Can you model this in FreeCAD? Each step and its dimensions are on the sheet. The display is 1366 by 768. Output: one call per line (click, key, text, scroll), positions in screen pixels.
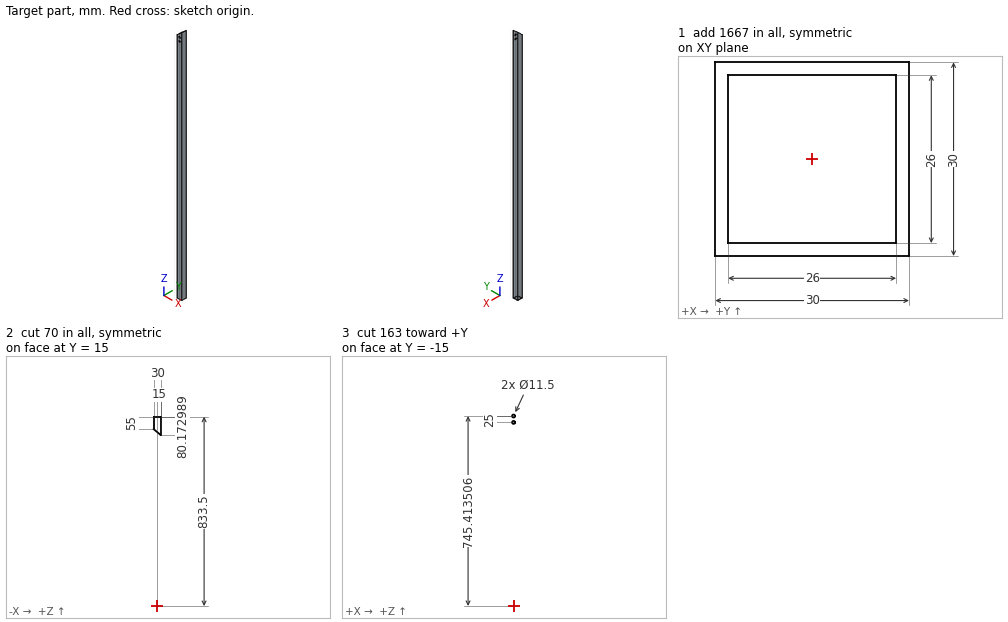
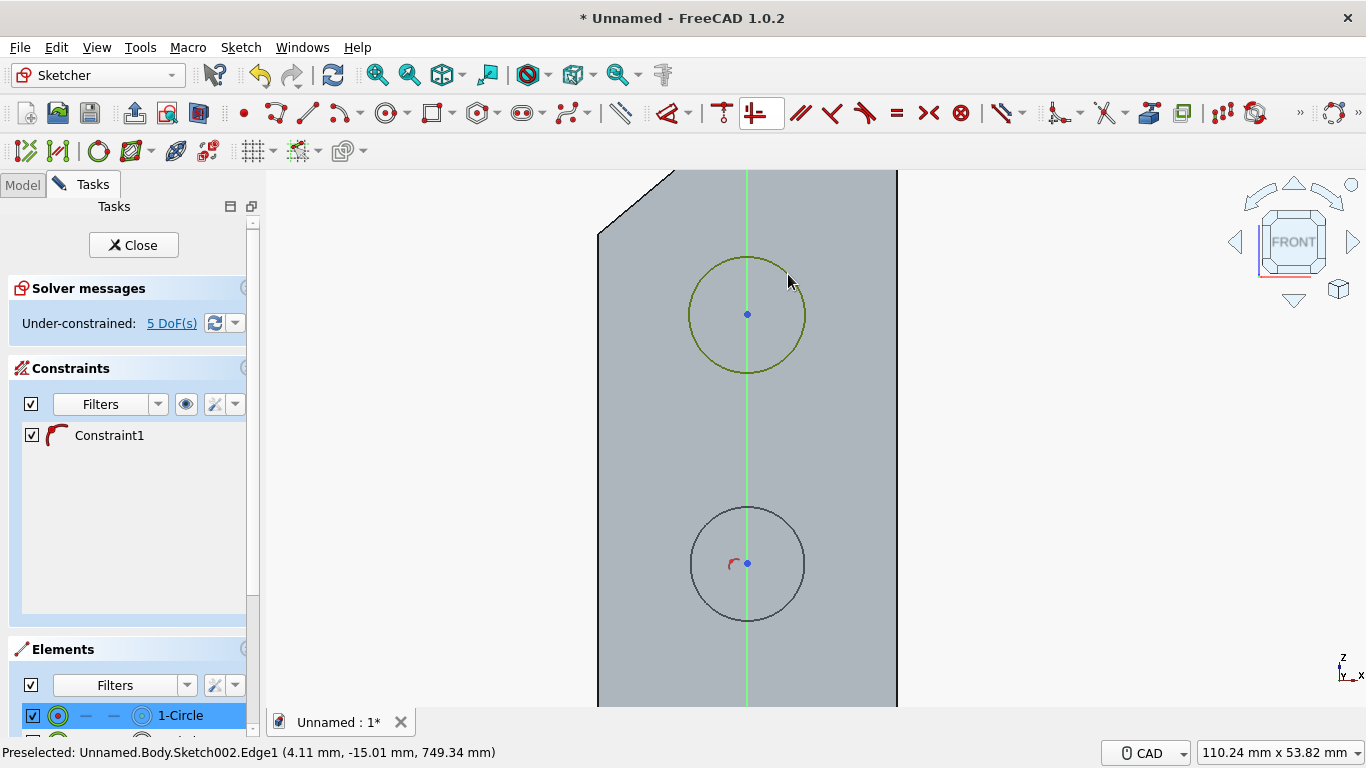
click(788, 524)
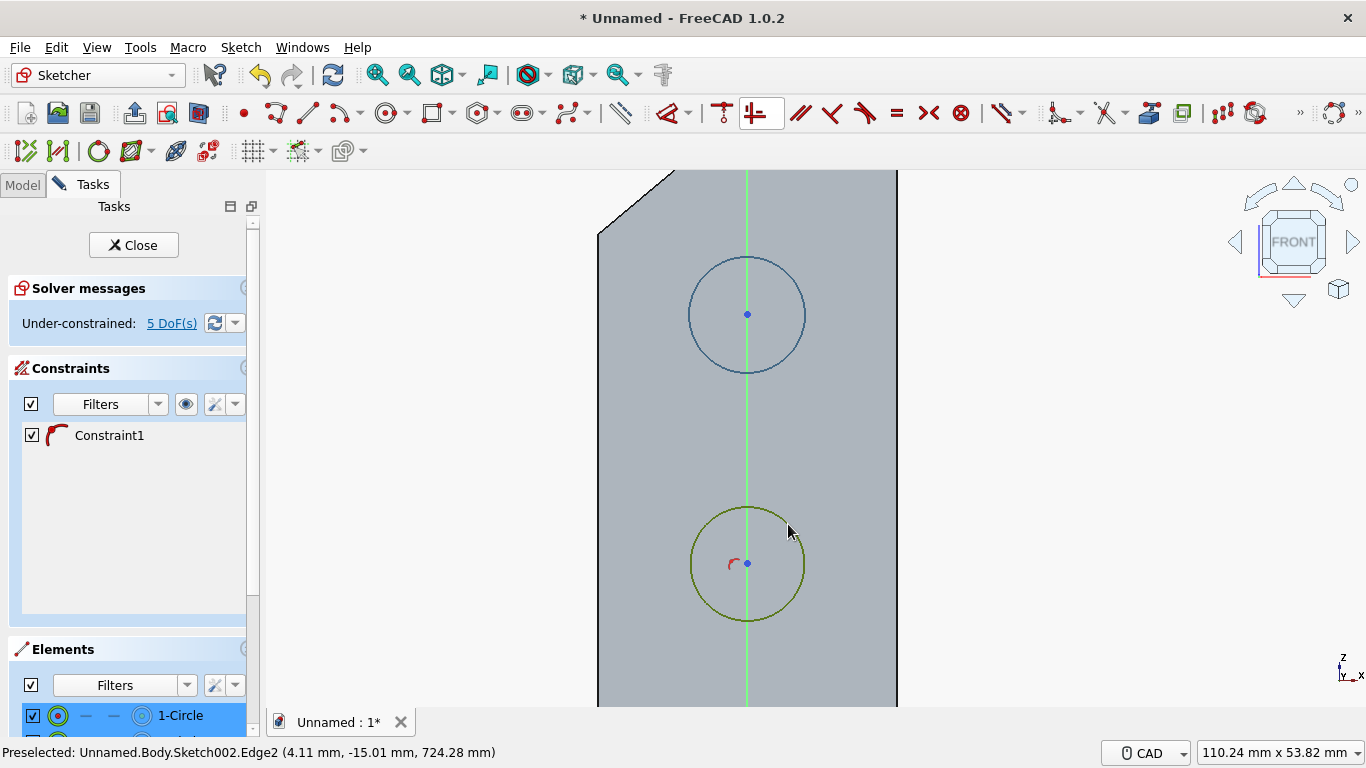
click(898, 114)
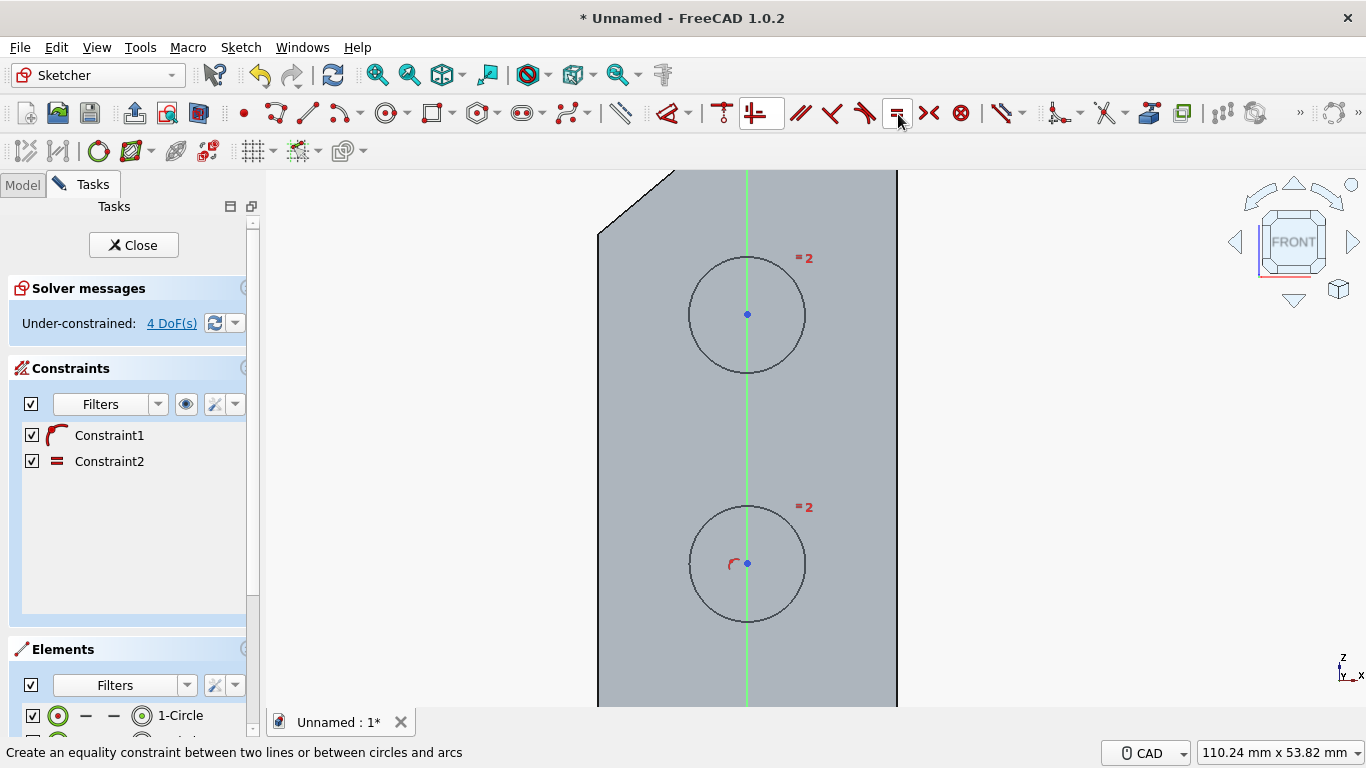
click(747, 315)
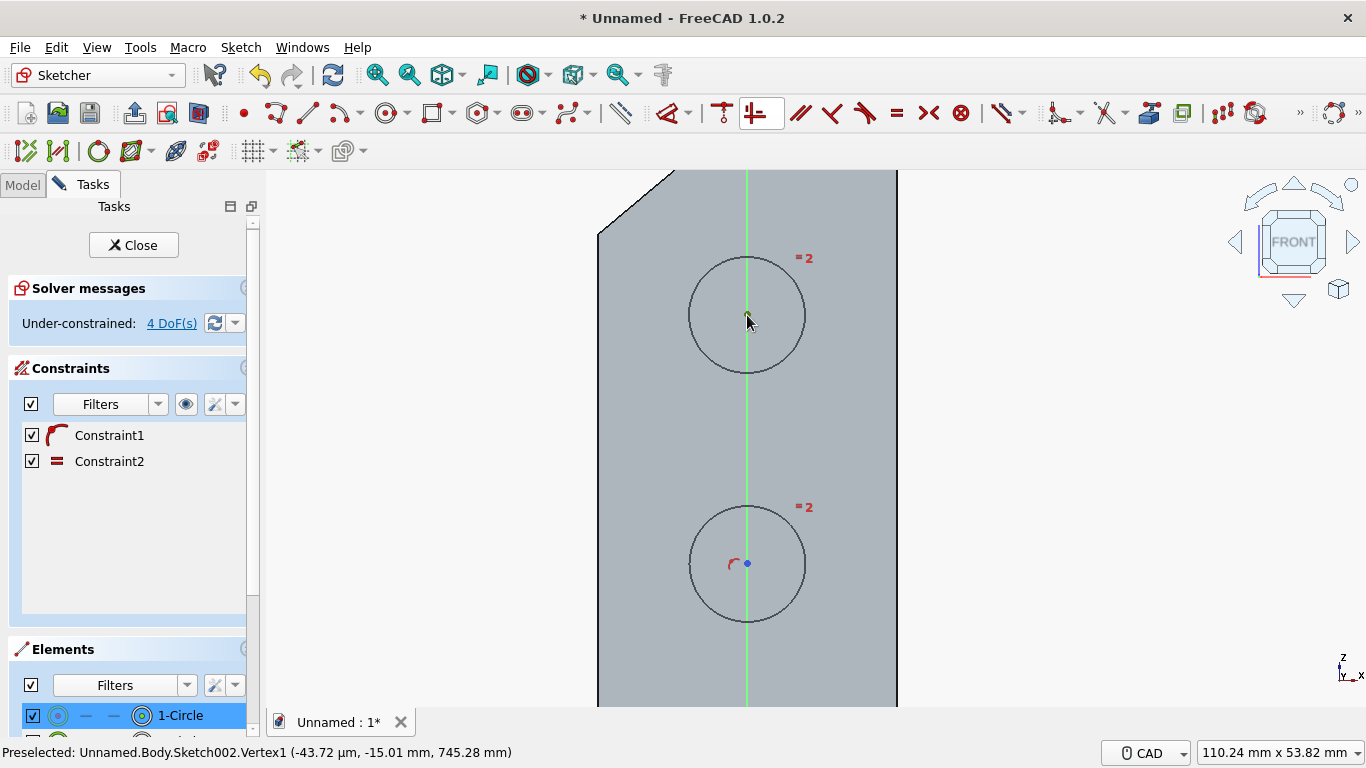
click(747, 576)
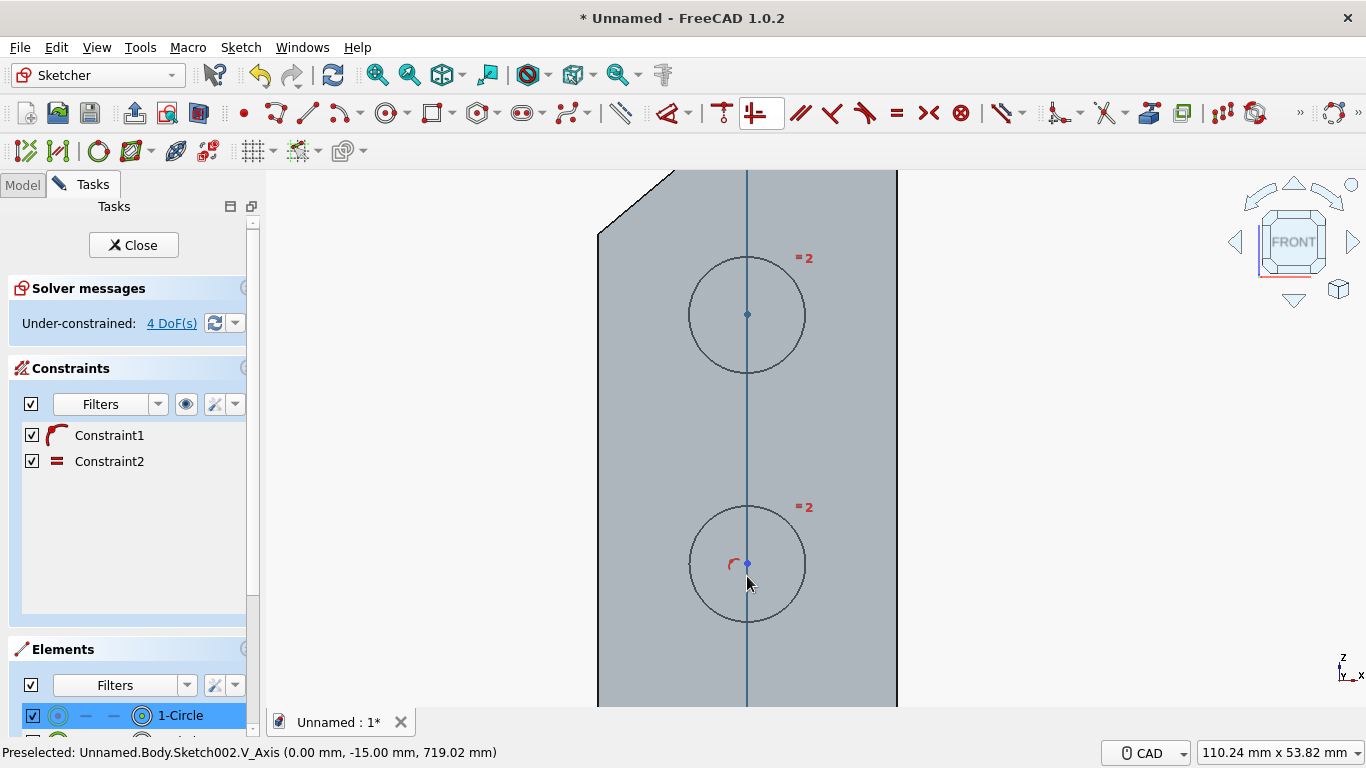
click(722, 114)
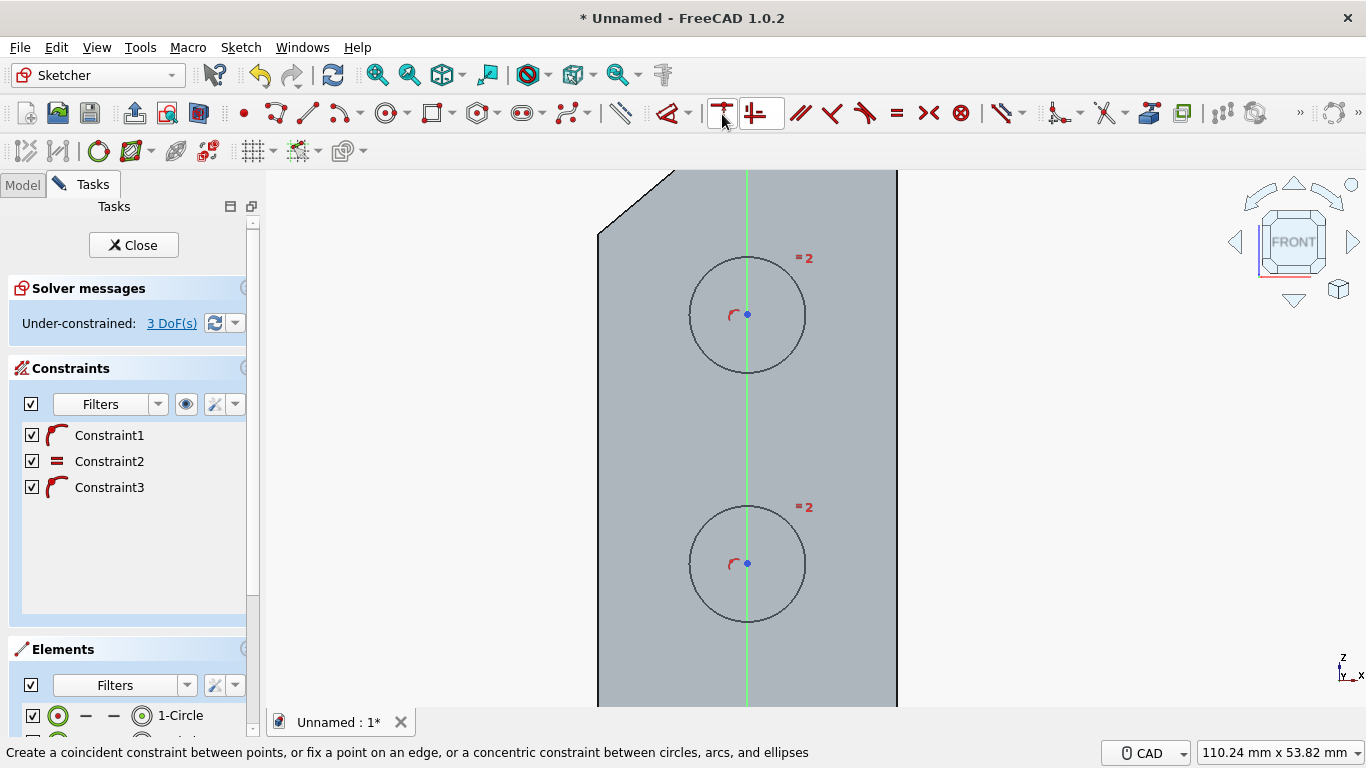
click(668, 114)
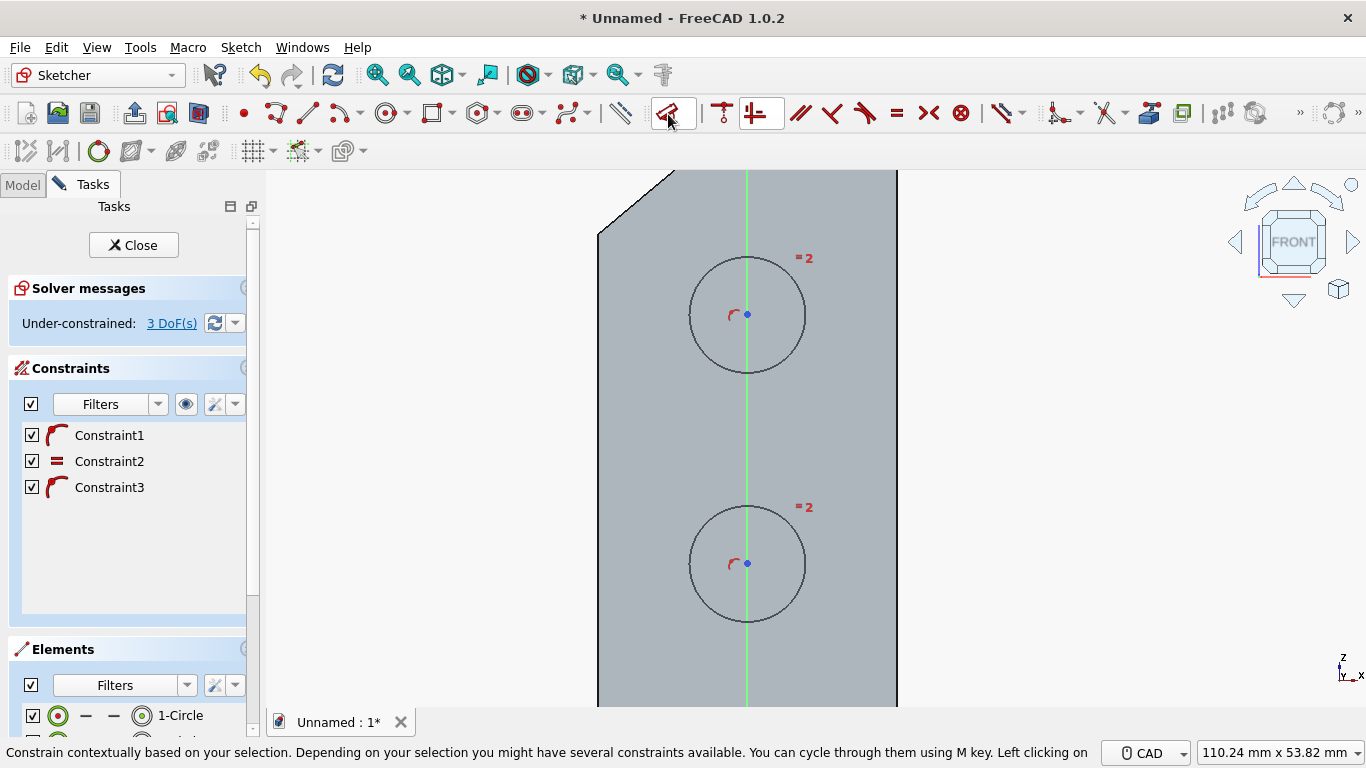
click(788, 274)
click(811, 251)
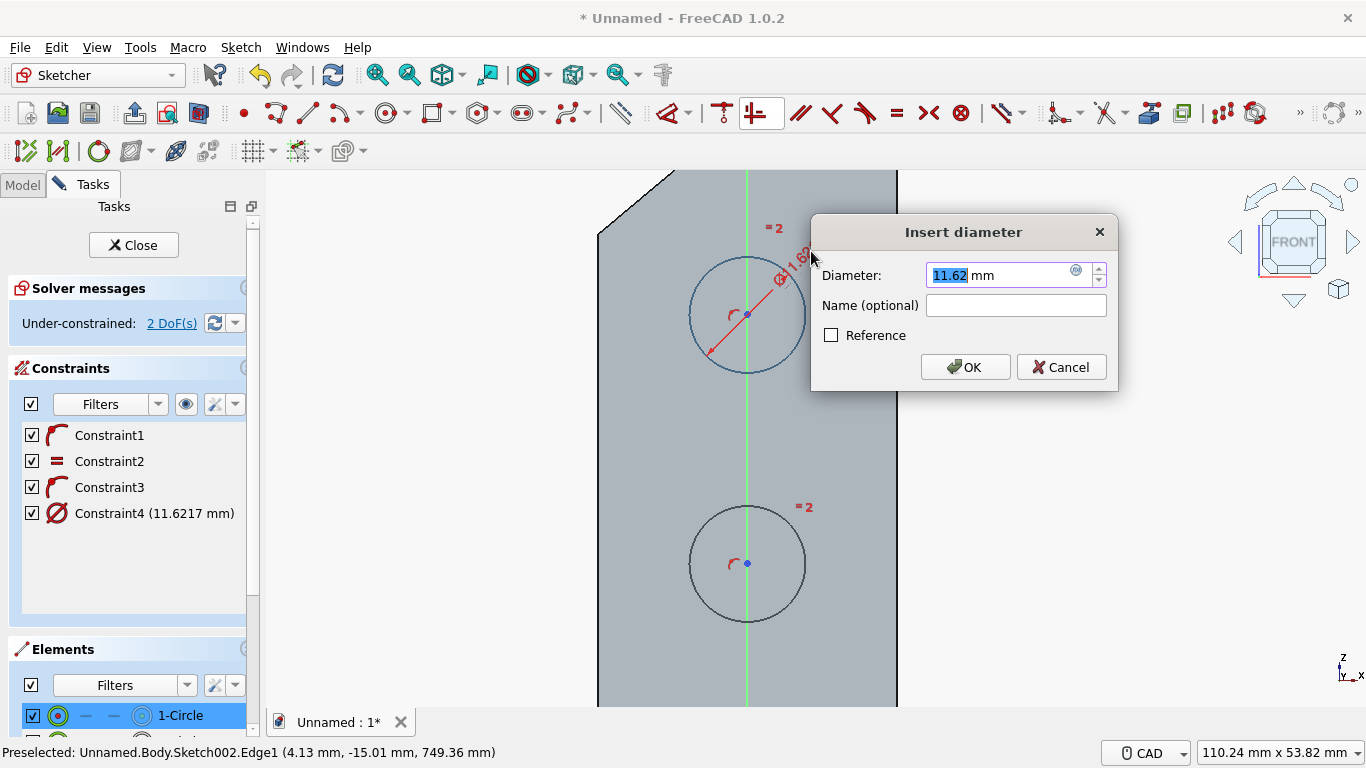
text(11.5)
key(Return)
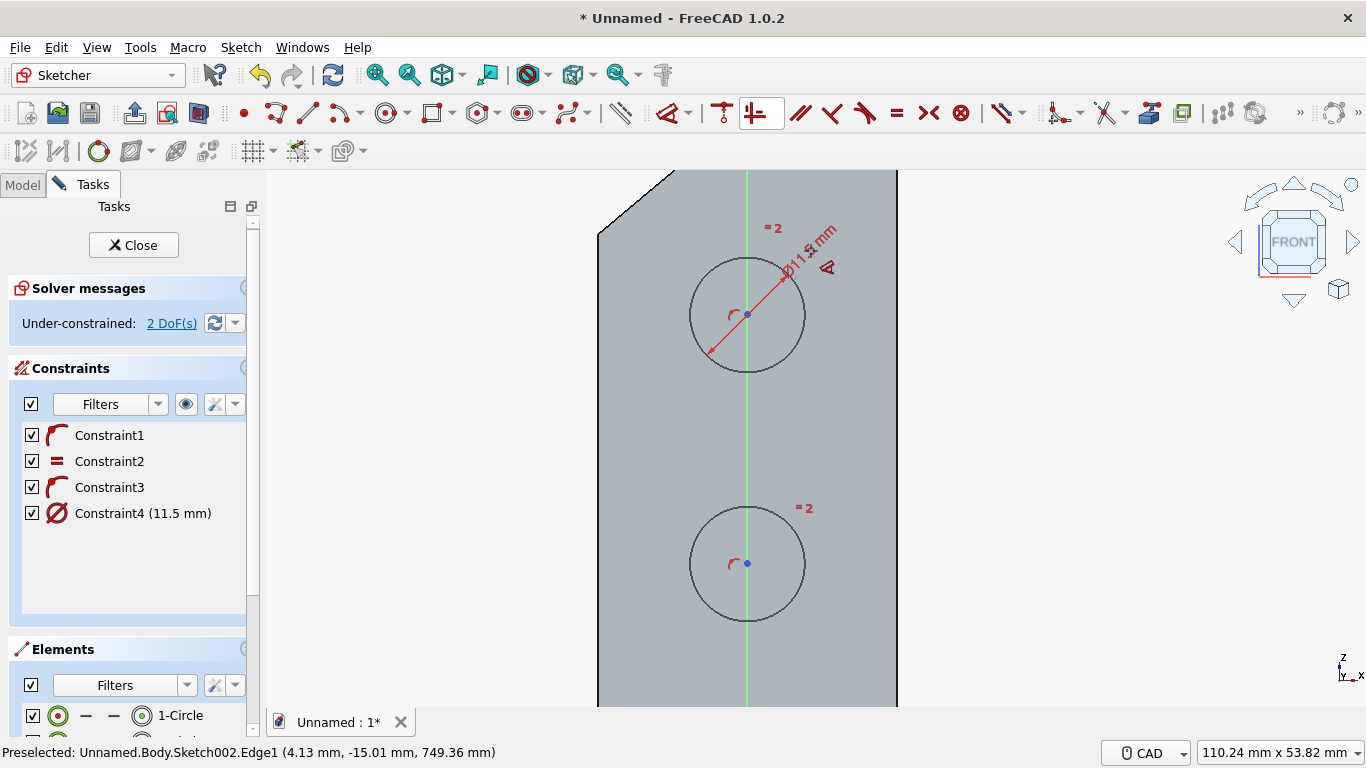
click(747, 315)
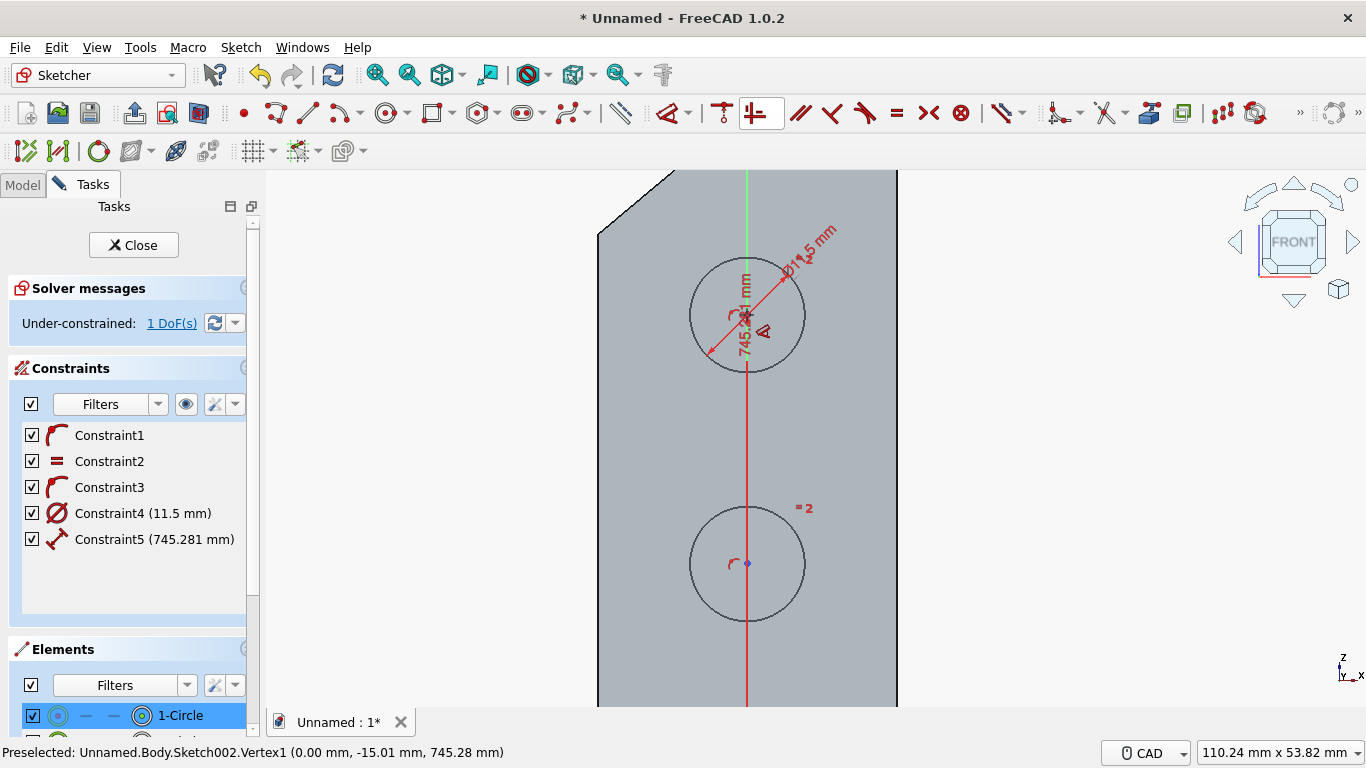
click(747, 564)
click(781, 440)